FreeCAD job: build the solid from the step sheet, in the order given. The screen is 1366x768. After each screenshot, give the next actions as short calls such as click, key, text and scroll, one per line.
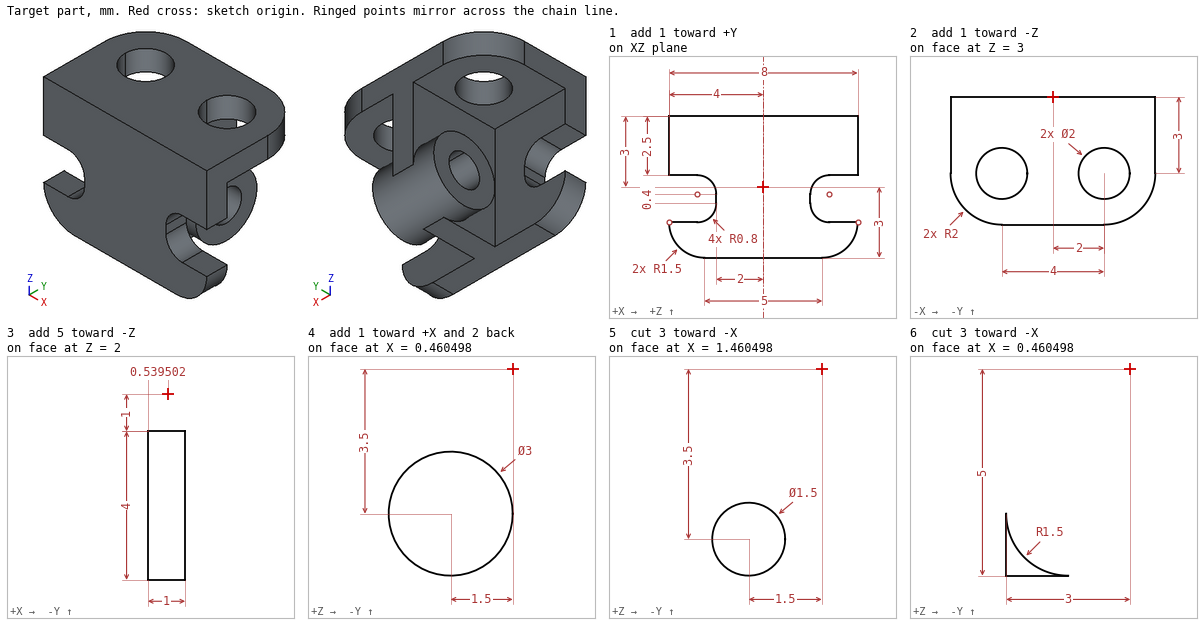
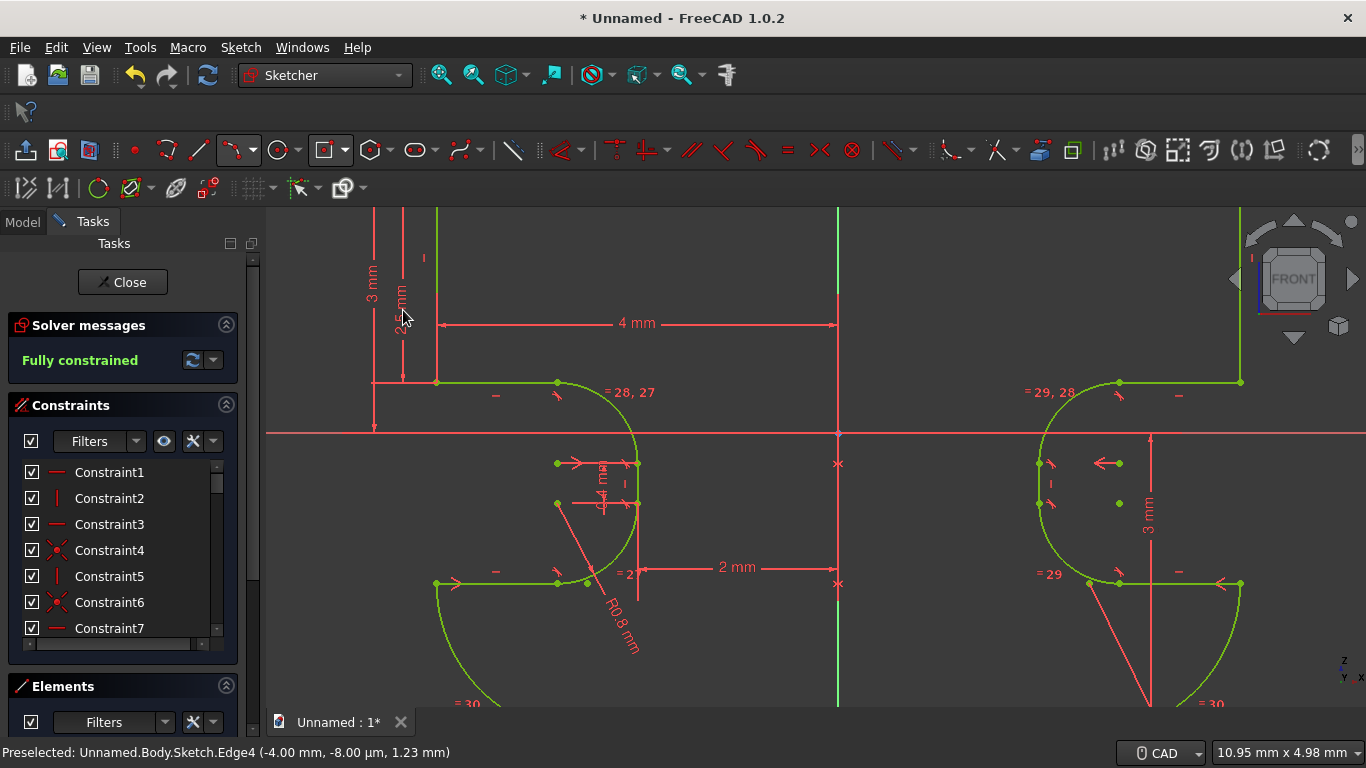
click(123, 282)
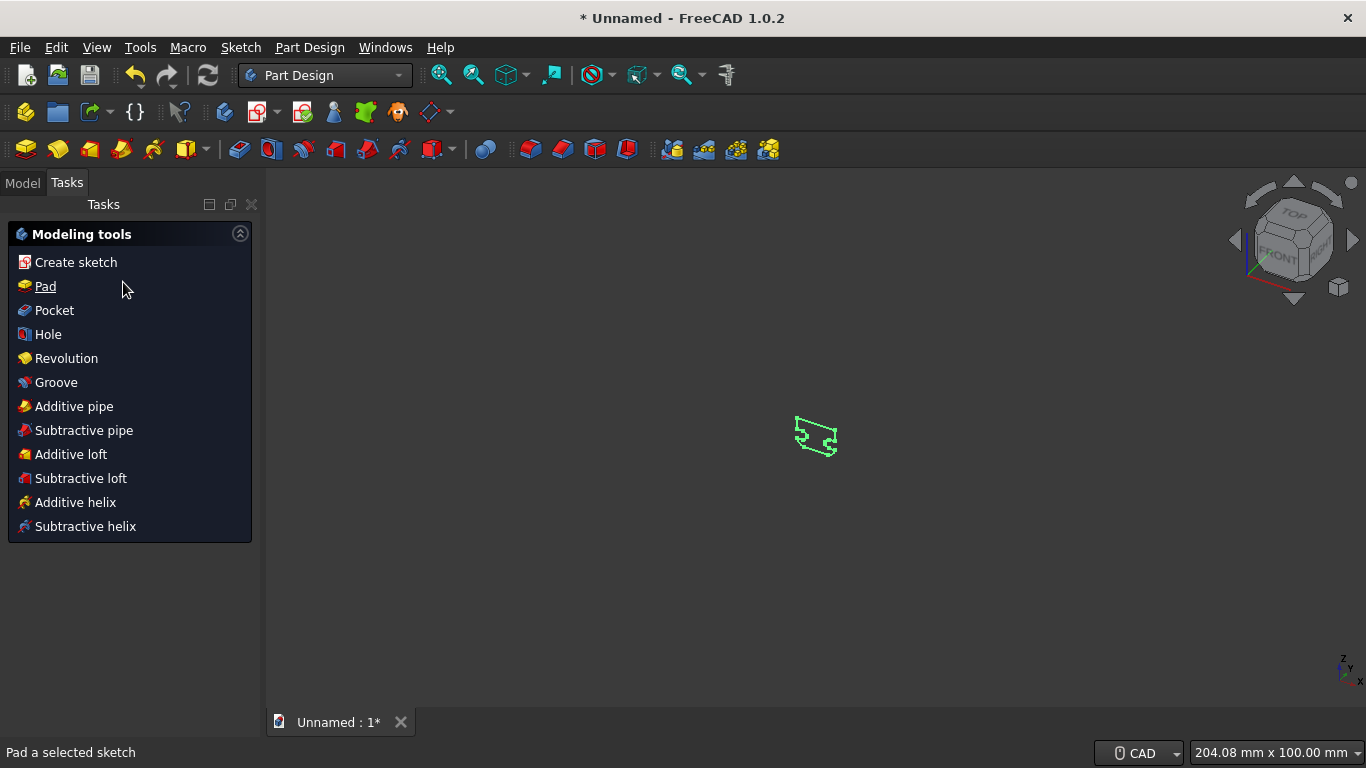
click(26, 150)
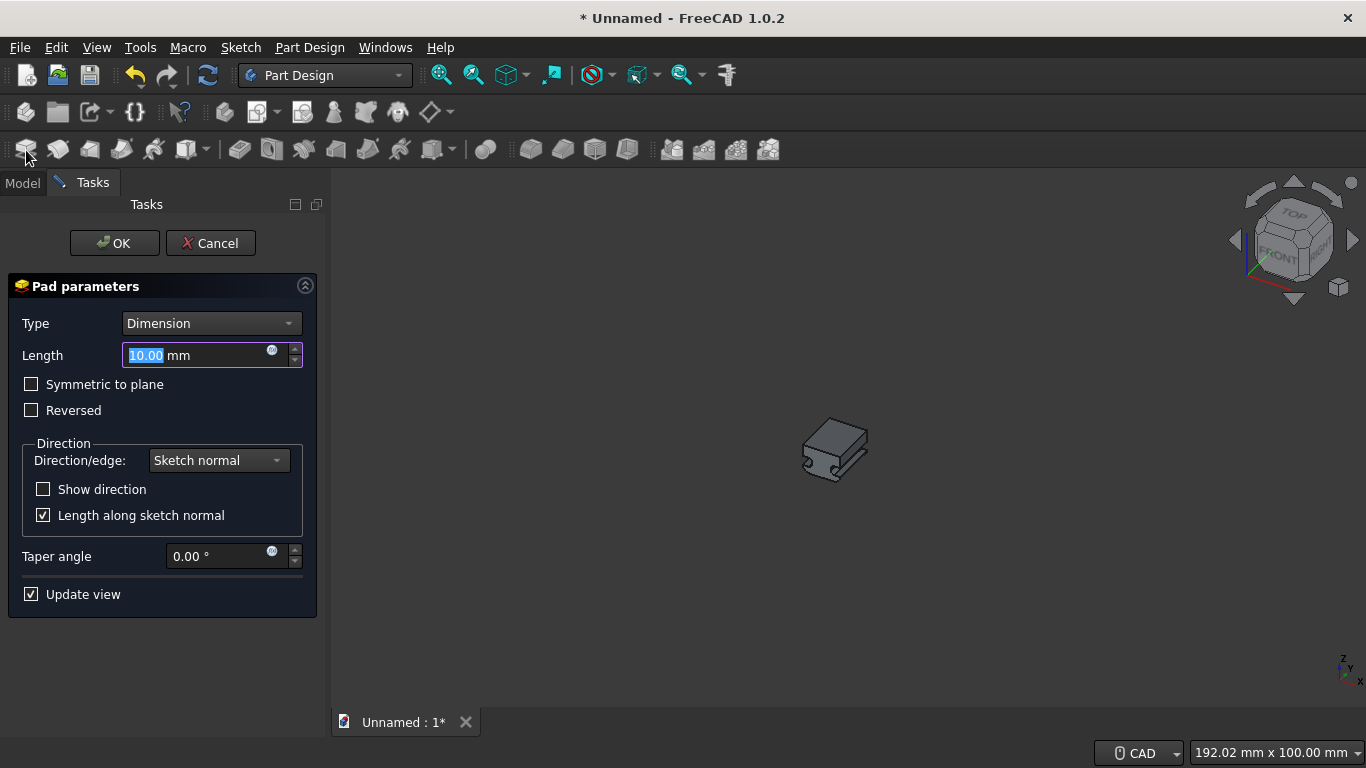
text(1)
key(Tab)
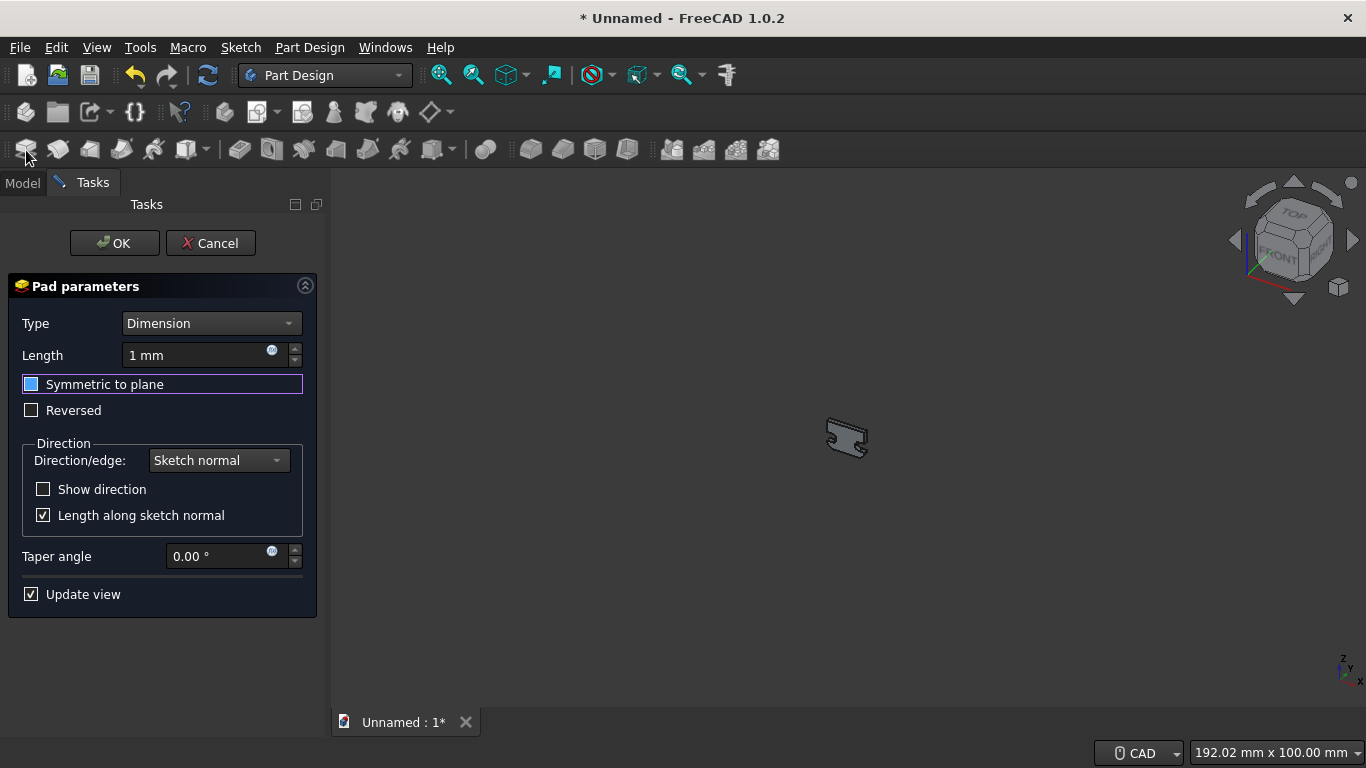
click(30, 410)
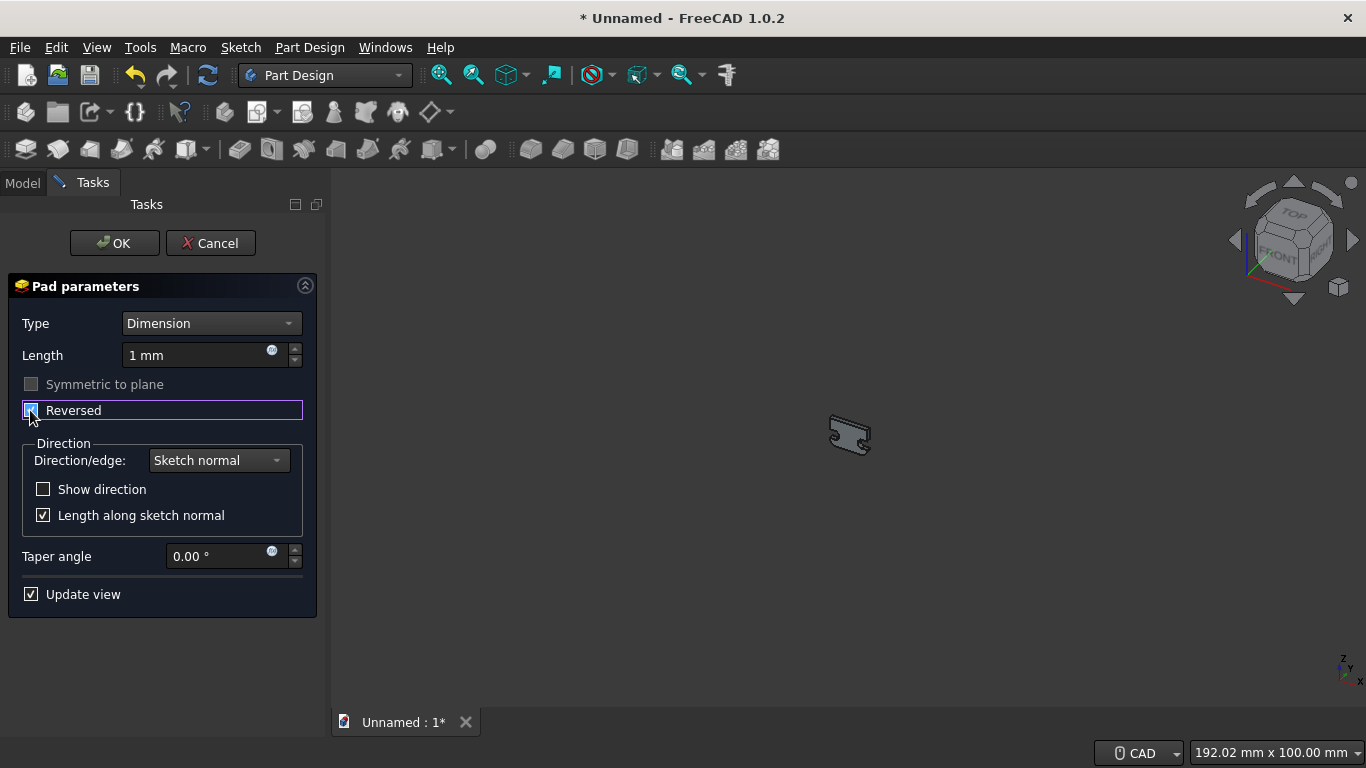
click(115, 243)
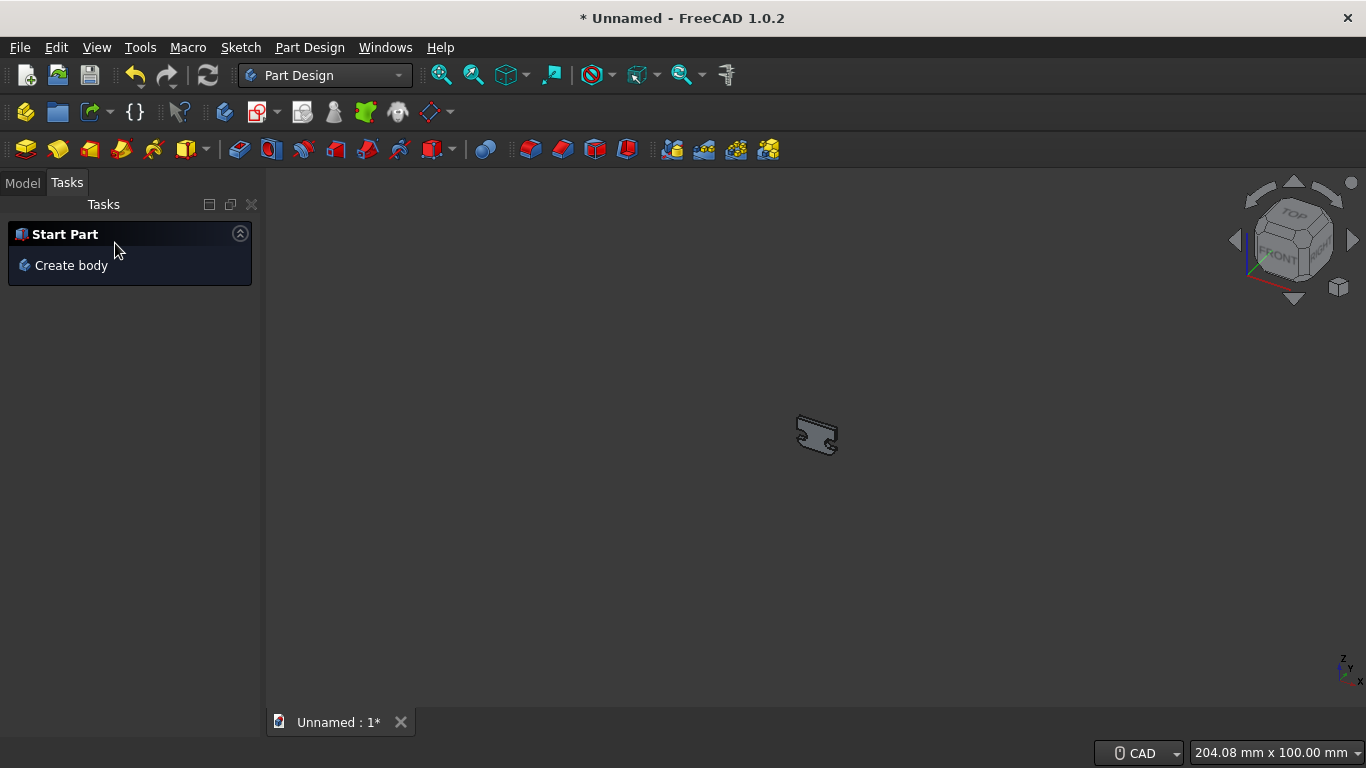
click(442, 76)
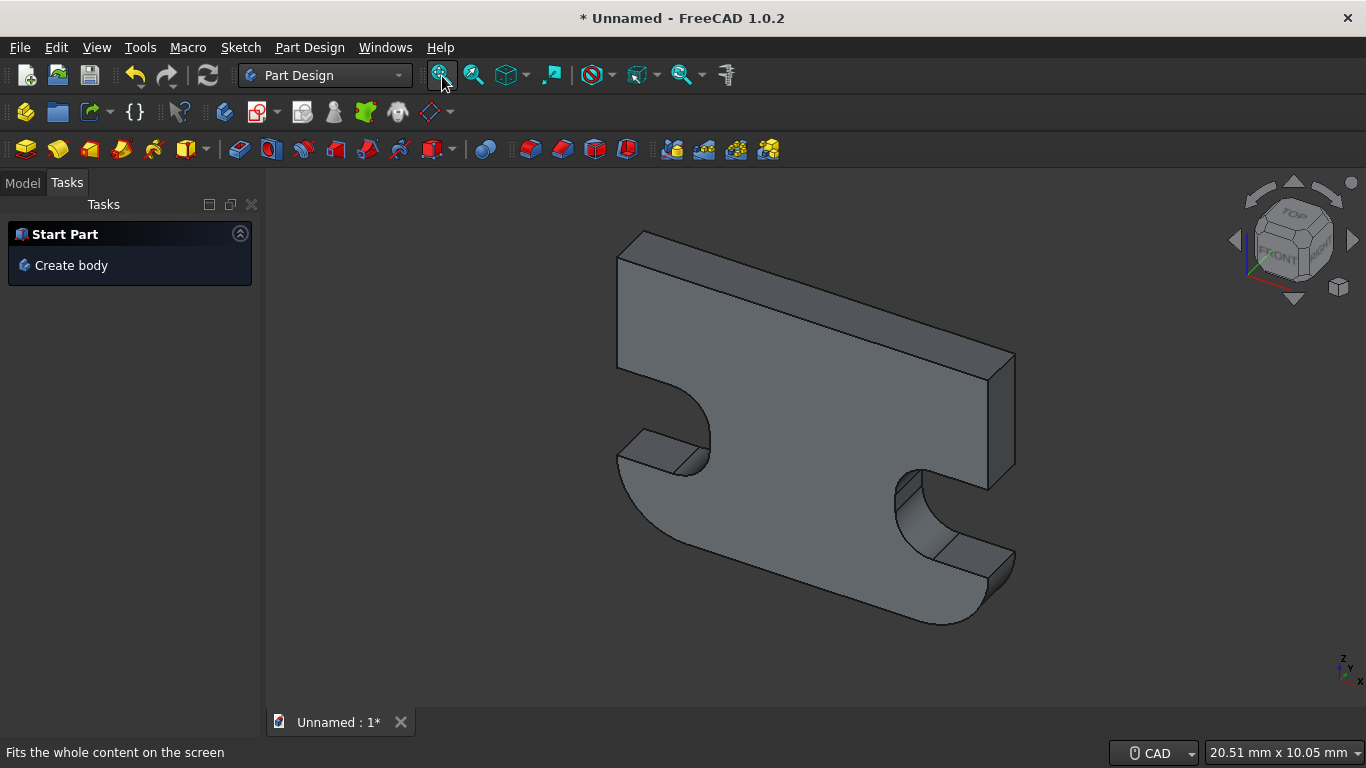
click(975, 357)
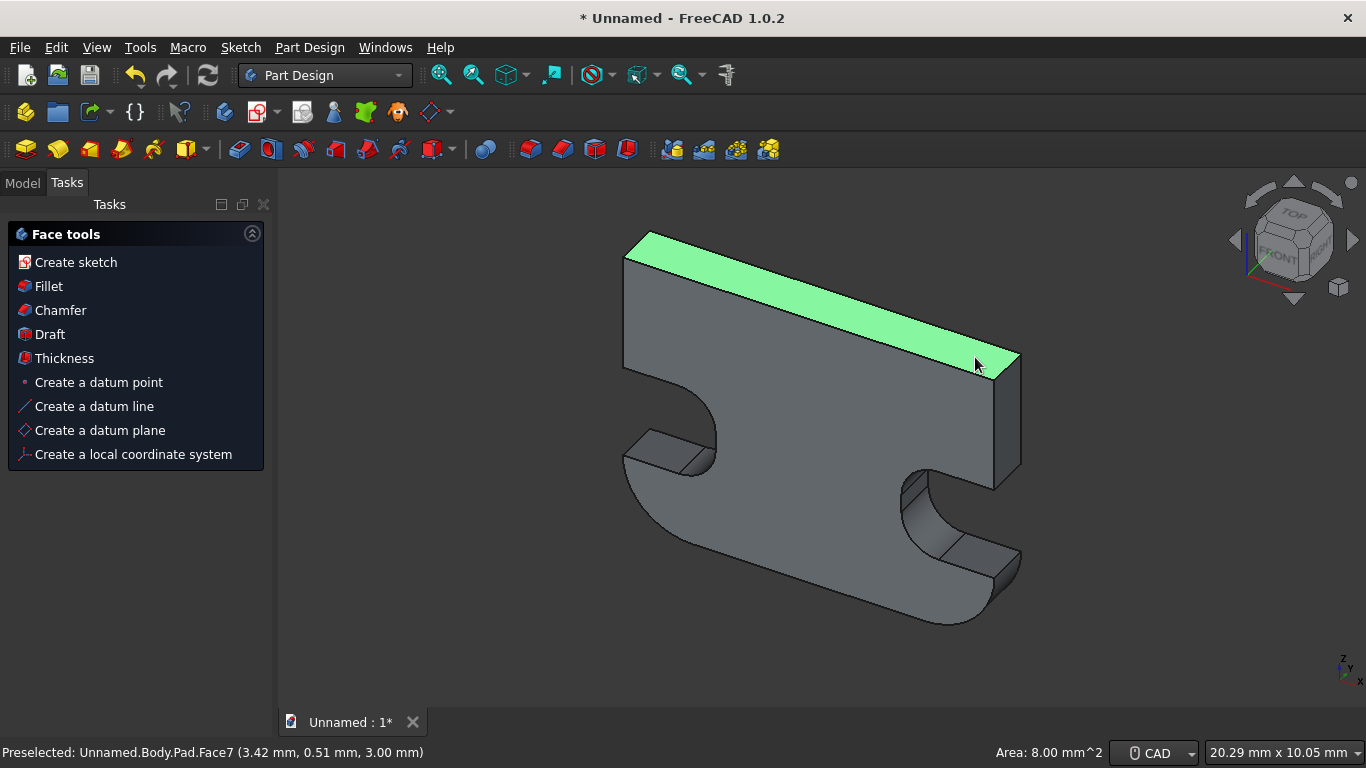
click(258, 112)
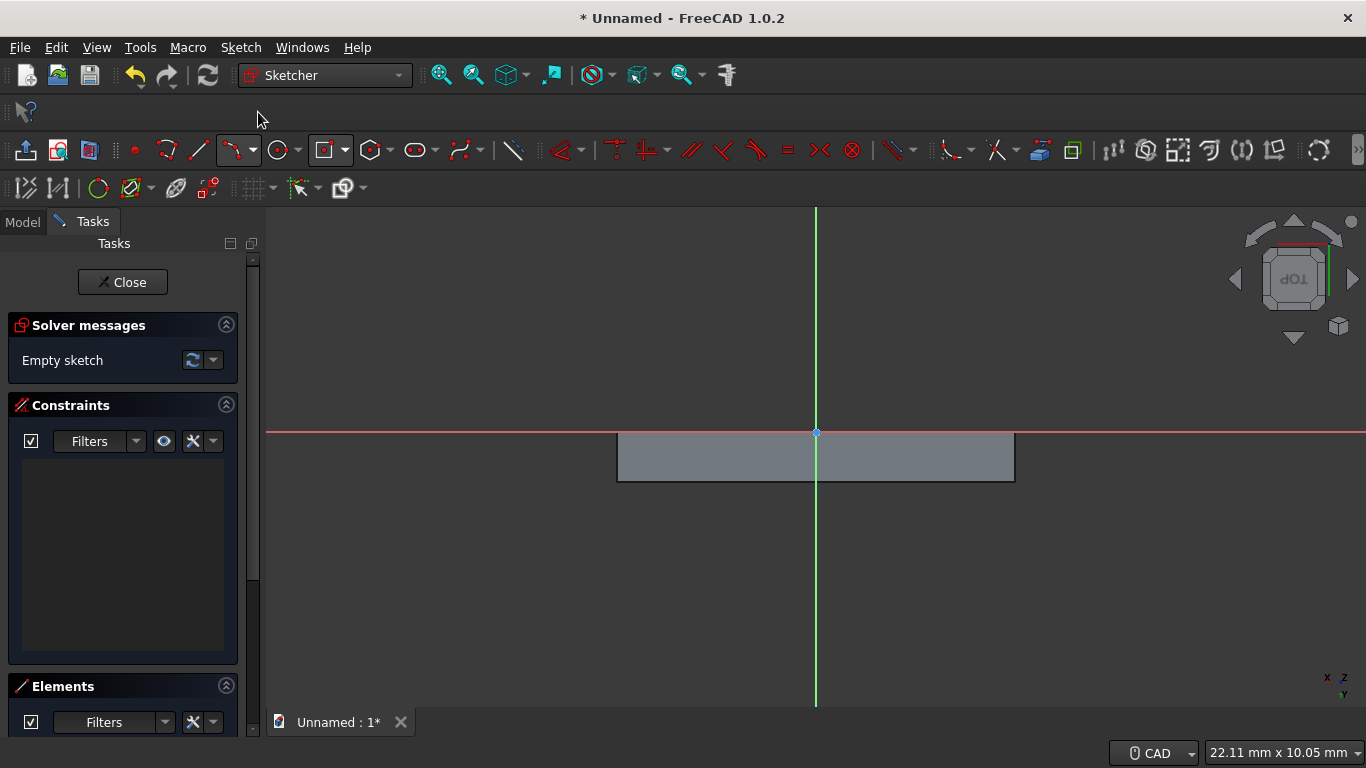
scroll(438, 235, down, 1)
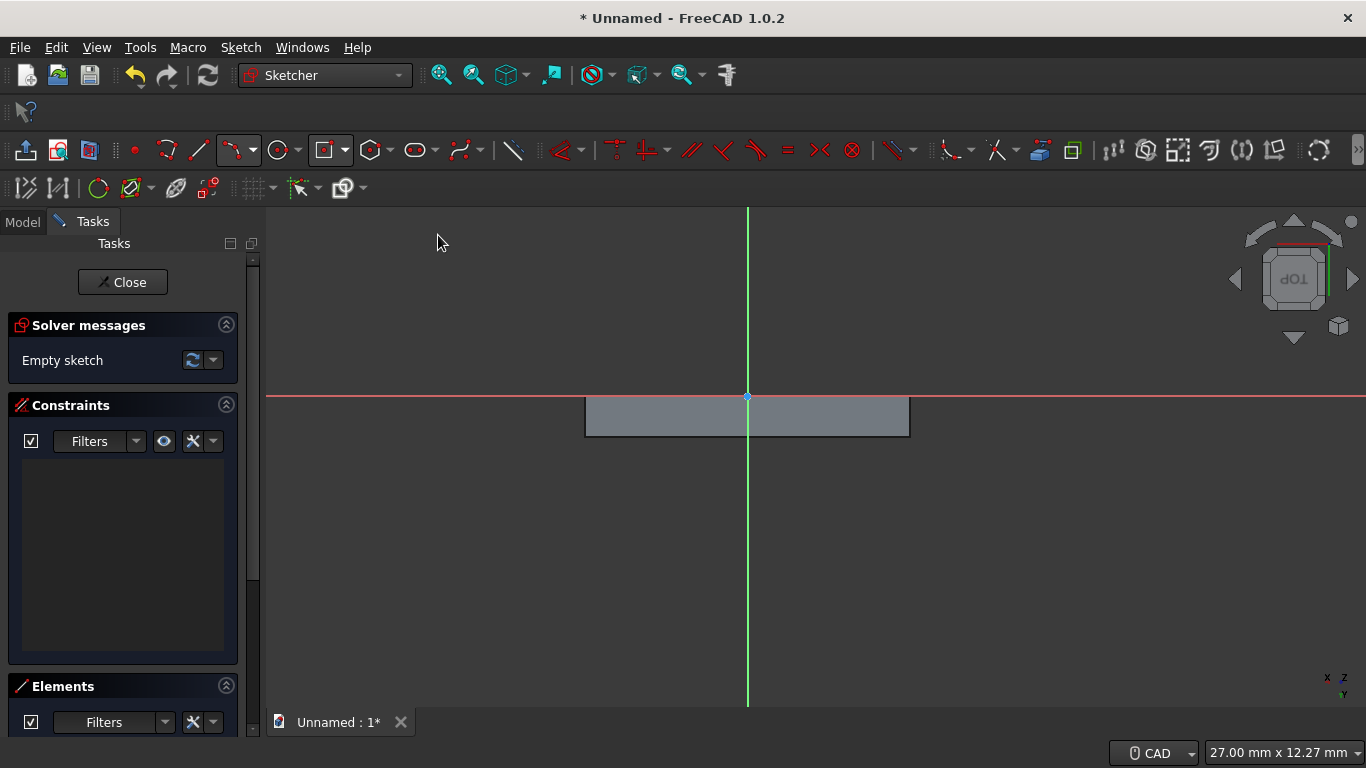
scroll(748, 582, up, 2)